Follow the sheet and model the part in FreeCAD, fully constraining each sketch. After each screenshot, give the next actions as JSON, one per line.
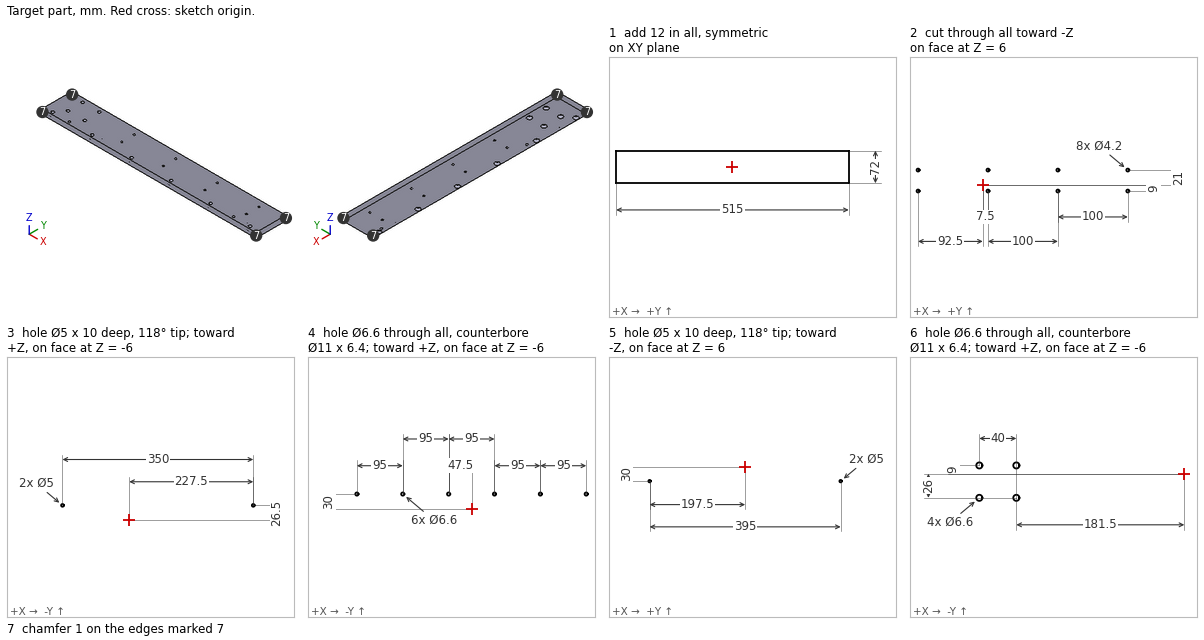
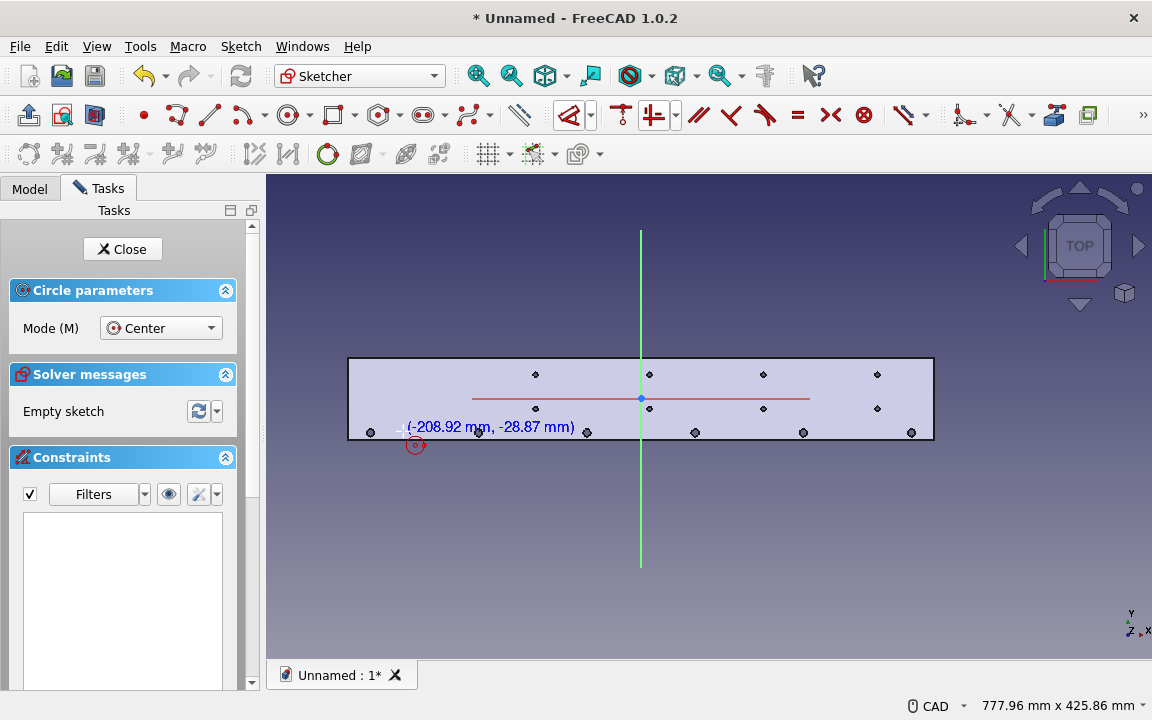
{"action": "left_click", "coordinate": [416, 433]}
{"action": "mouse_move", "coordinate": [418, 431]}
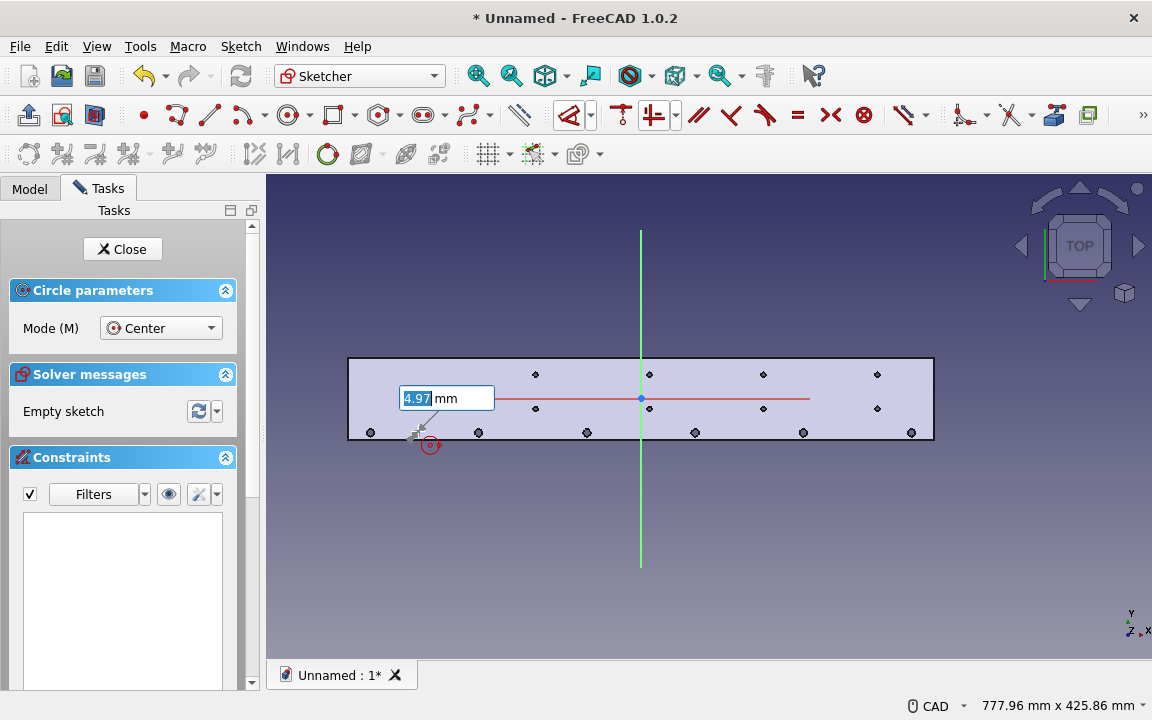
{"action": "type", "text": "5"}
{"action": "key", "text": "Return"}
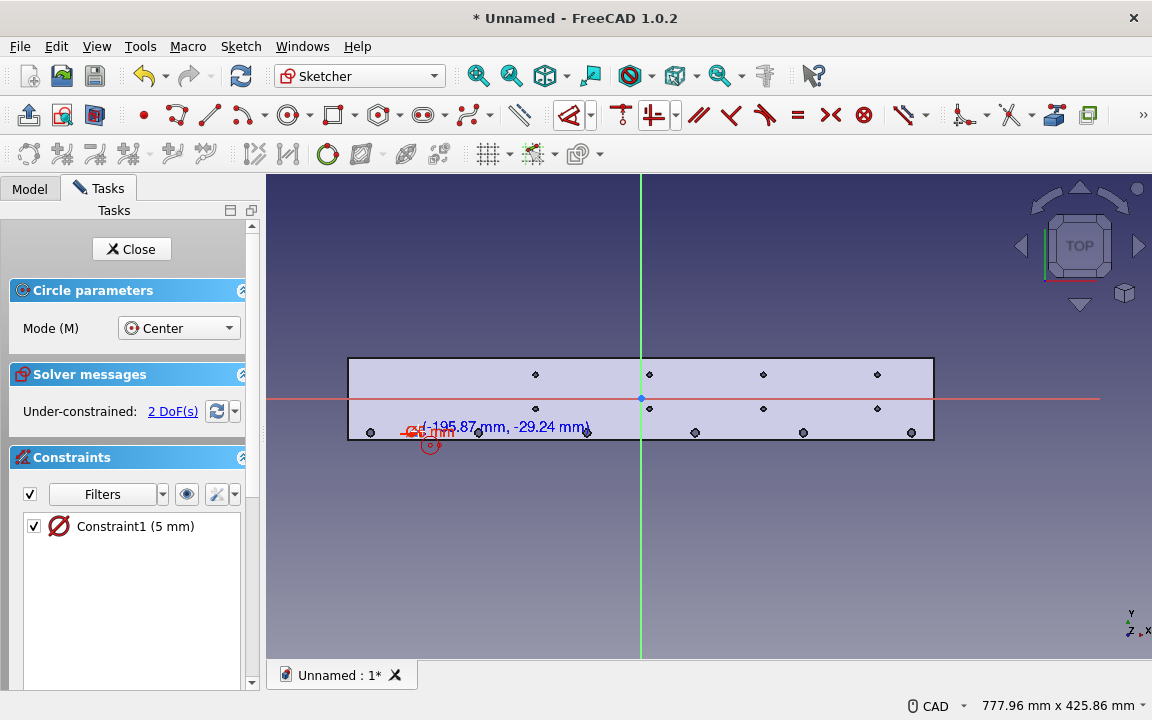
{"action": "scroll", "coordinate": [866, 433], "scroll_direction": "up", "scroll_amount": 11}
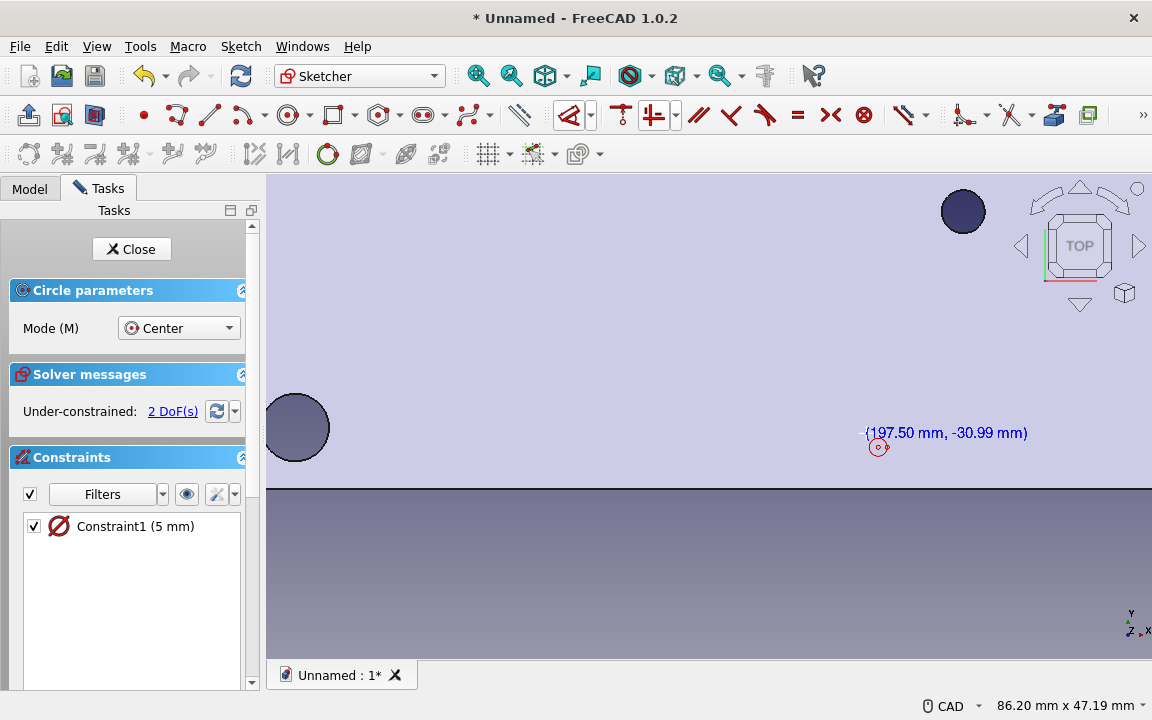
{"action": "scroll", "coordinate": [866, 433], "scroll_direction": "down", "scroll_amount": 11}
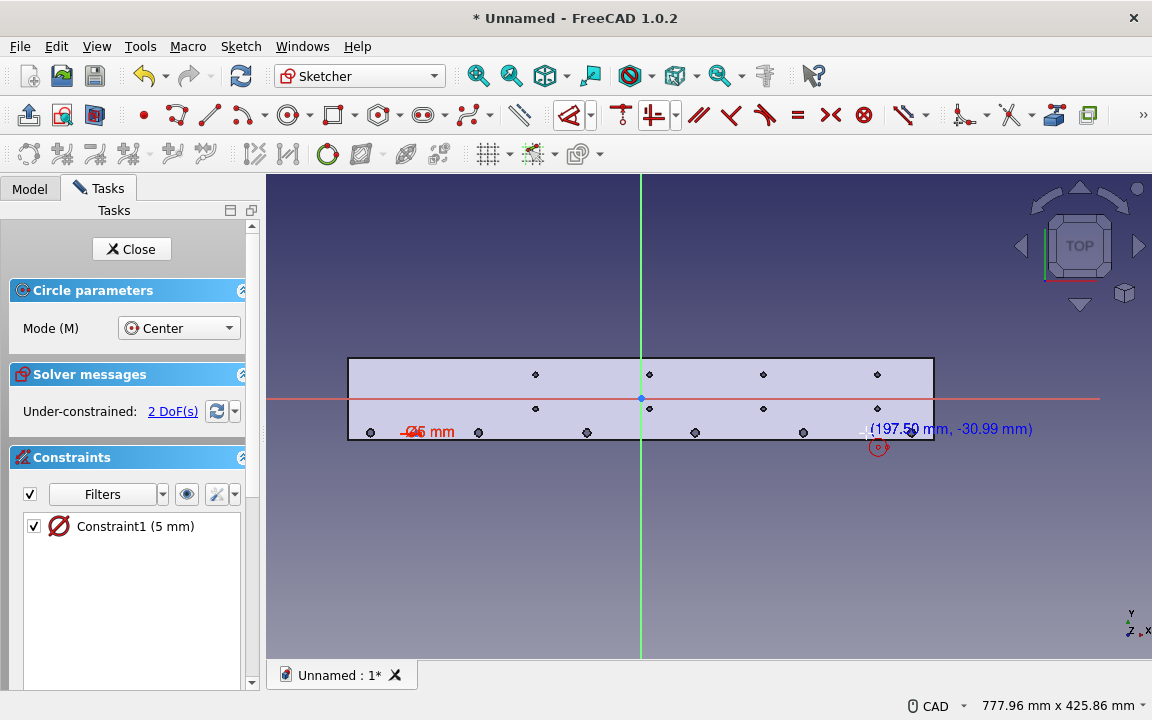
{"action": "left_click", "coordinate": [866, 433]}
{"action": "mouse_move", "coordinate": [868, 431]}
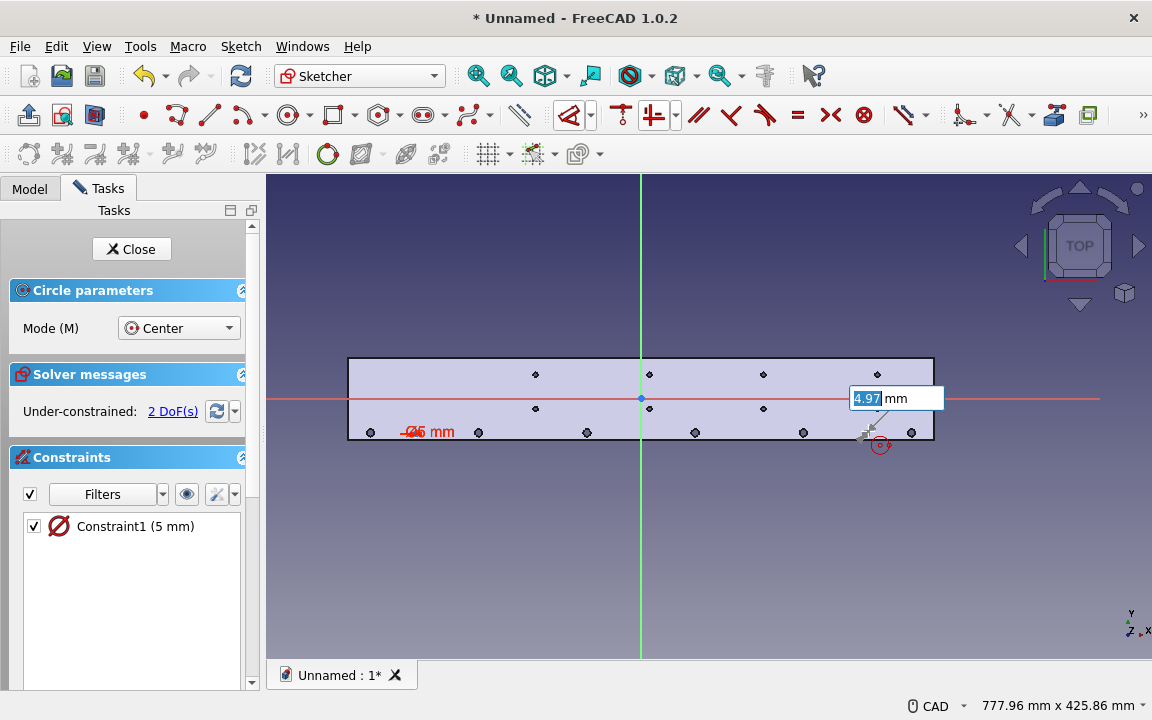
{"action": "type", "text": "5"}
{"action": "key", "text": "Return"}
{"action": "key", "text": "Escape"}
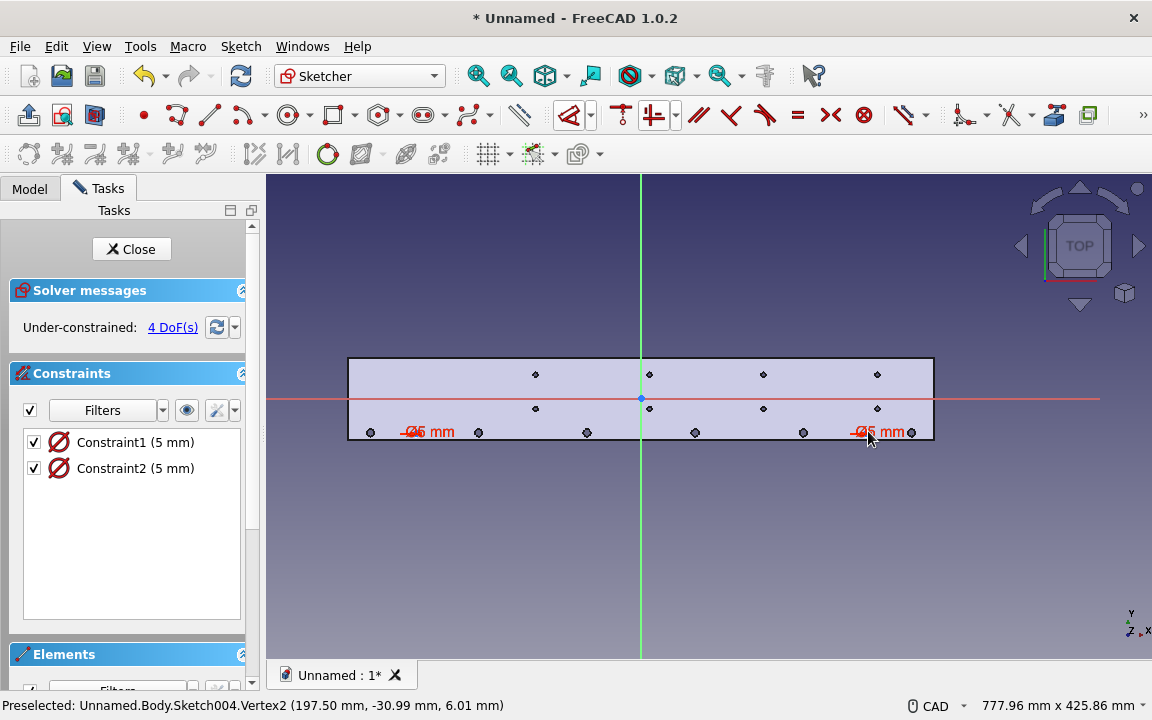
{"action": "left_click", "coordinate": [416, 434]}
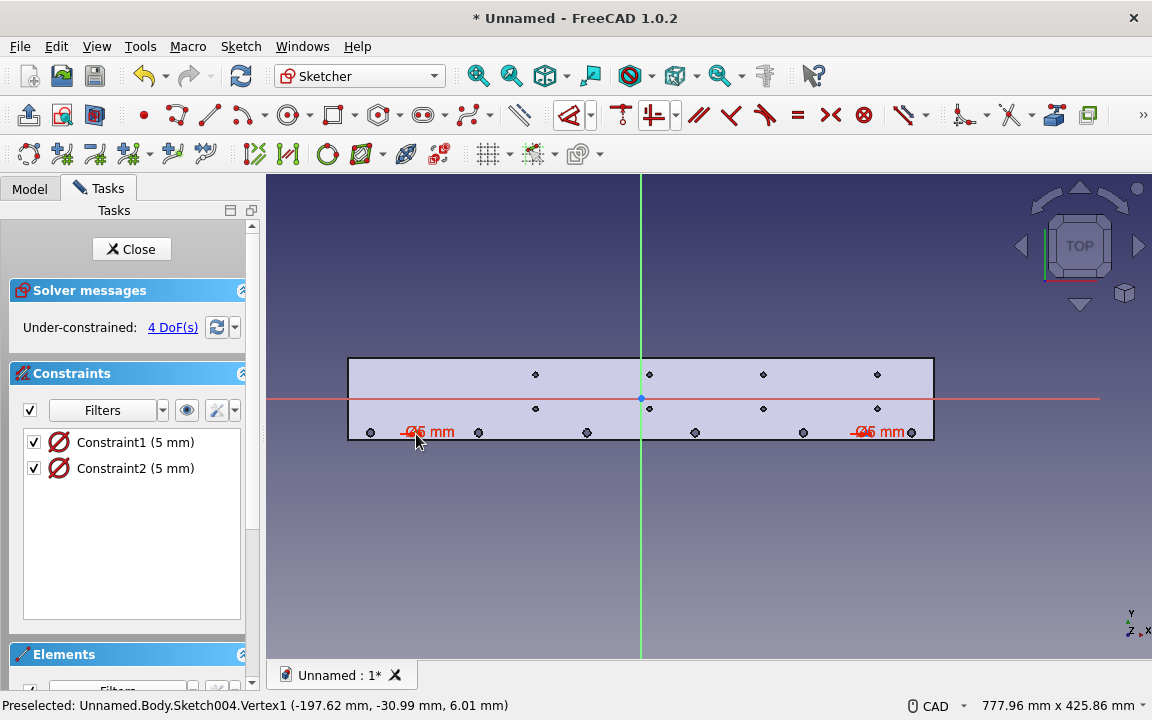
{"action": "left_click", "coordinate": [866, 434]}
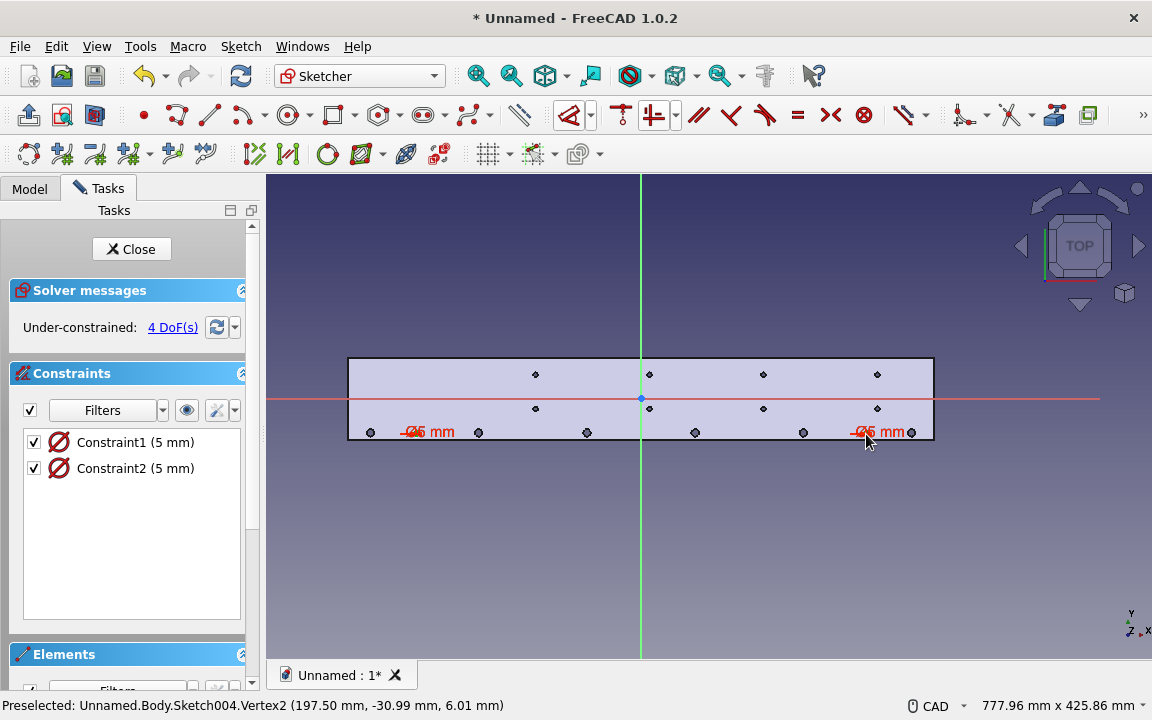
{"action": "left_click", "coordinate": [676, 116]}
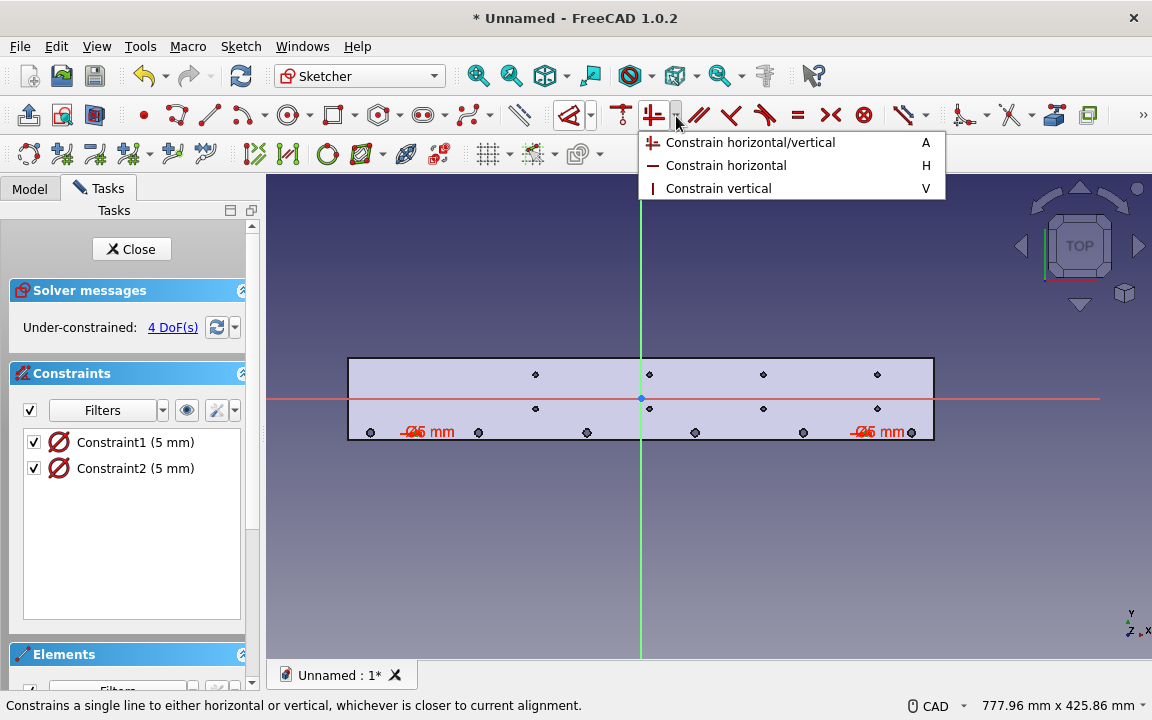
{"action": "left_click", "coordinate": [792, 166]}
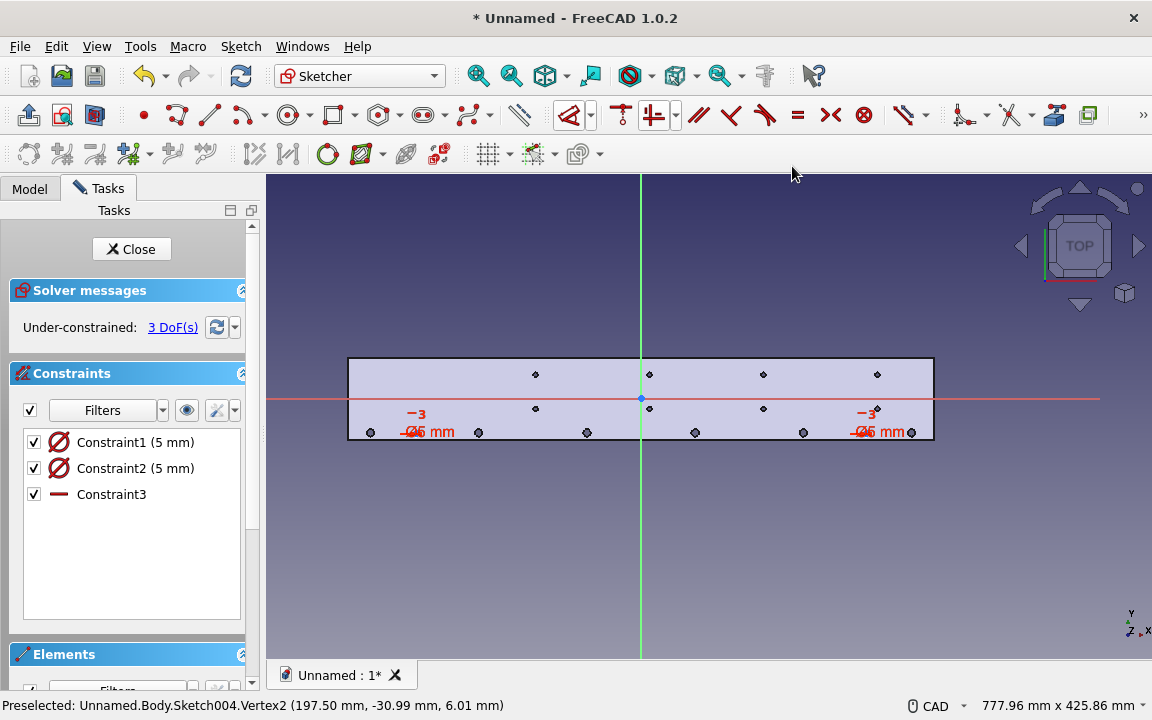
{"action": "left_click", "coordinate": [416, 434]}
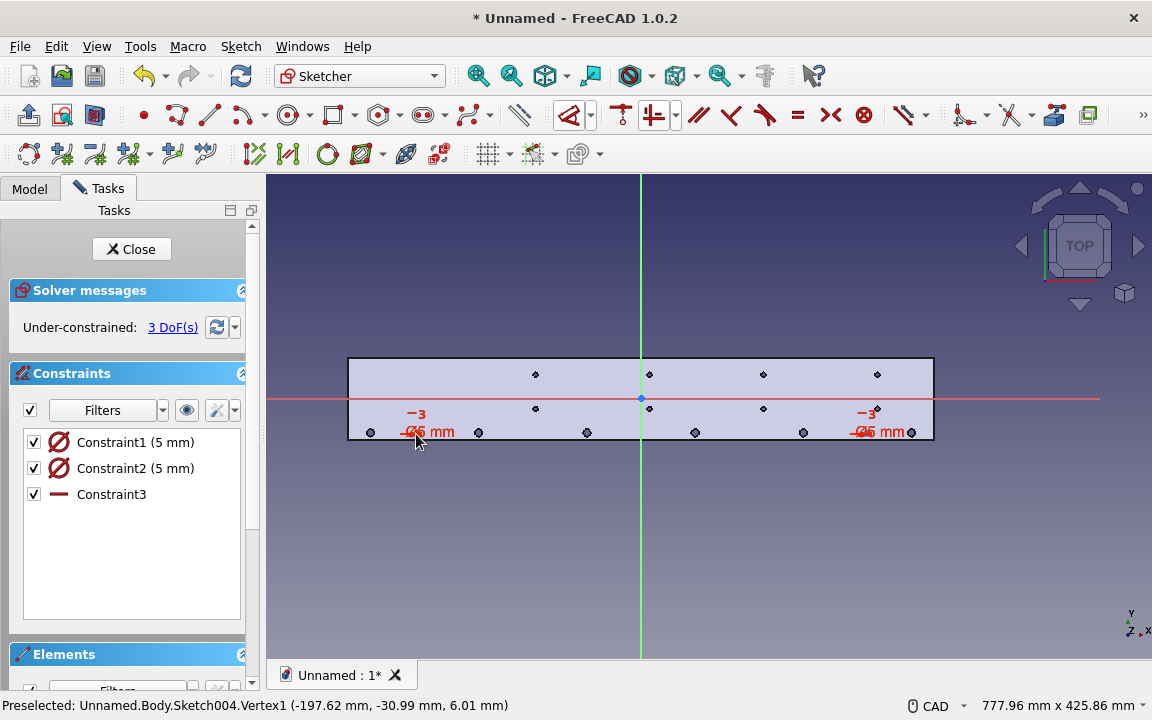
{"action": "key", "text": "i"}